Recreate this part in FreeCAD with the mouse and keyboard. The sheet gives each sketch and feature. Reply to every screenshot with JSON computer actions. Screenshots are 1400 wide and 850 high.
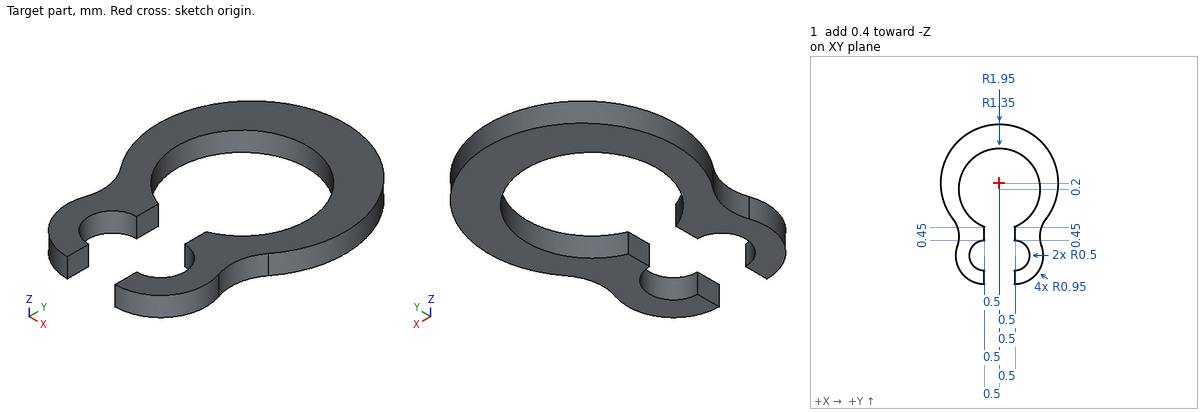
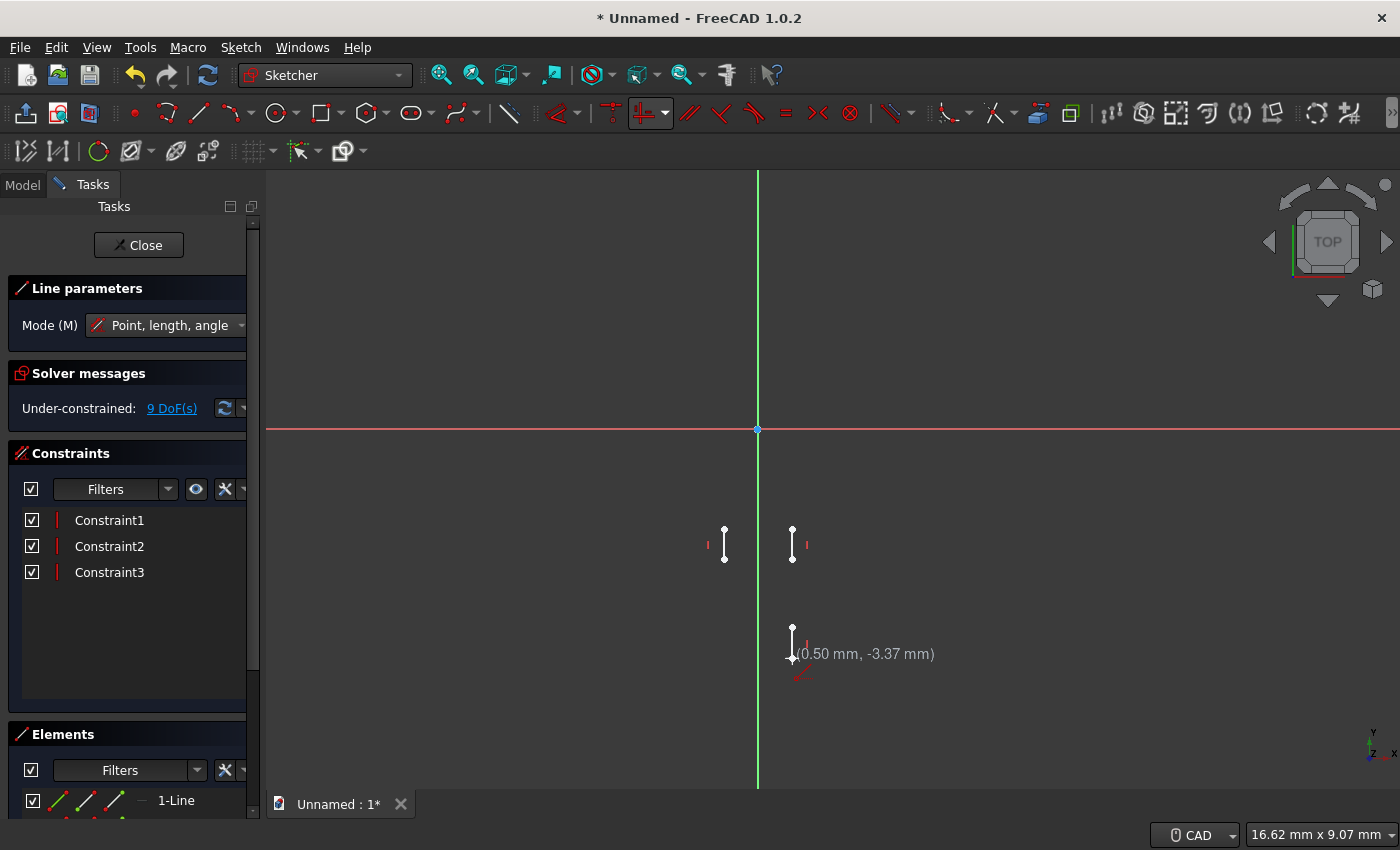
{"action": "left_click", "coordinate": [724, 658]}
{"action": "left_click", "coordinate": [724, 627]}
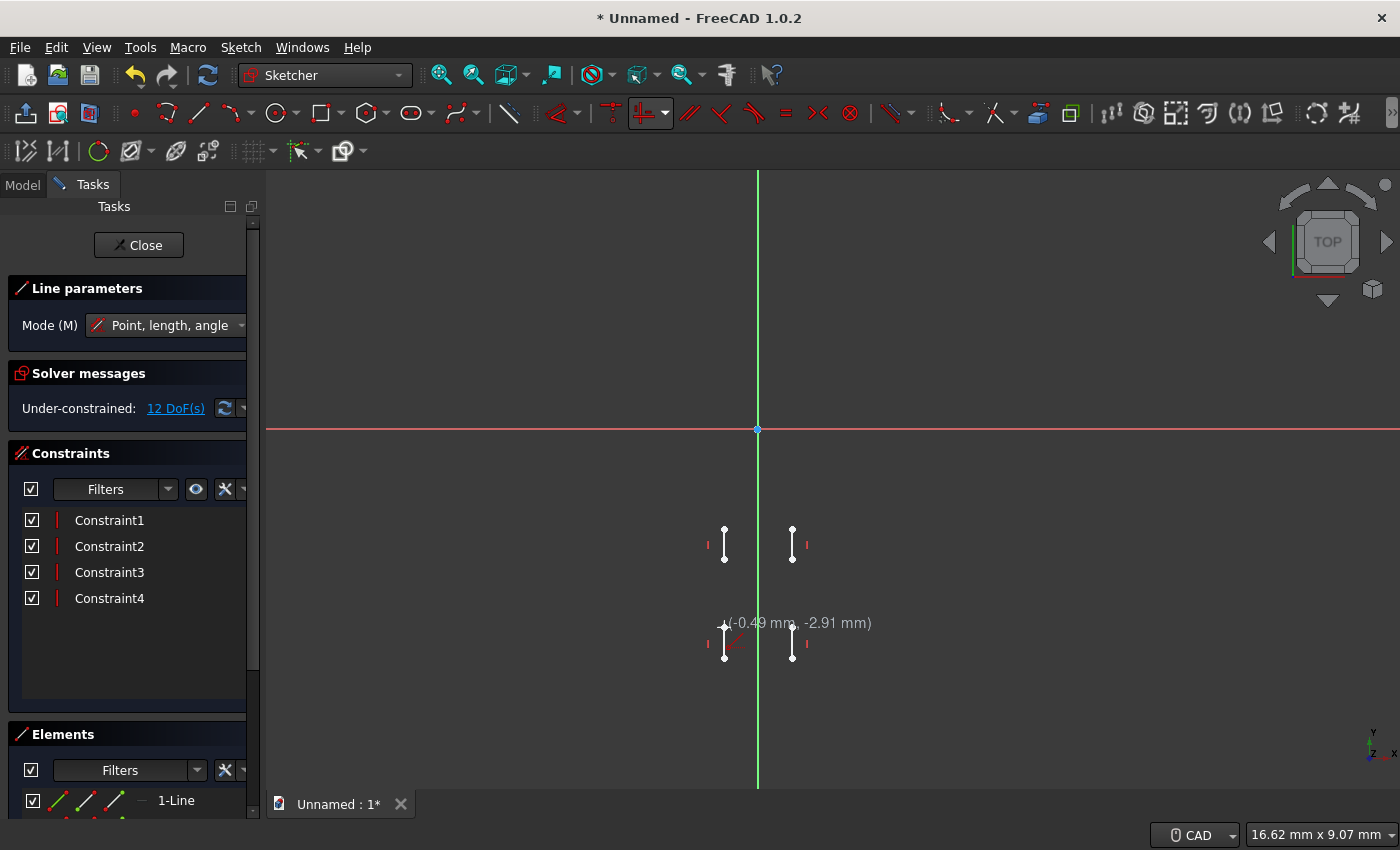
{"action": "left_click", "coordinate": [232, 114]}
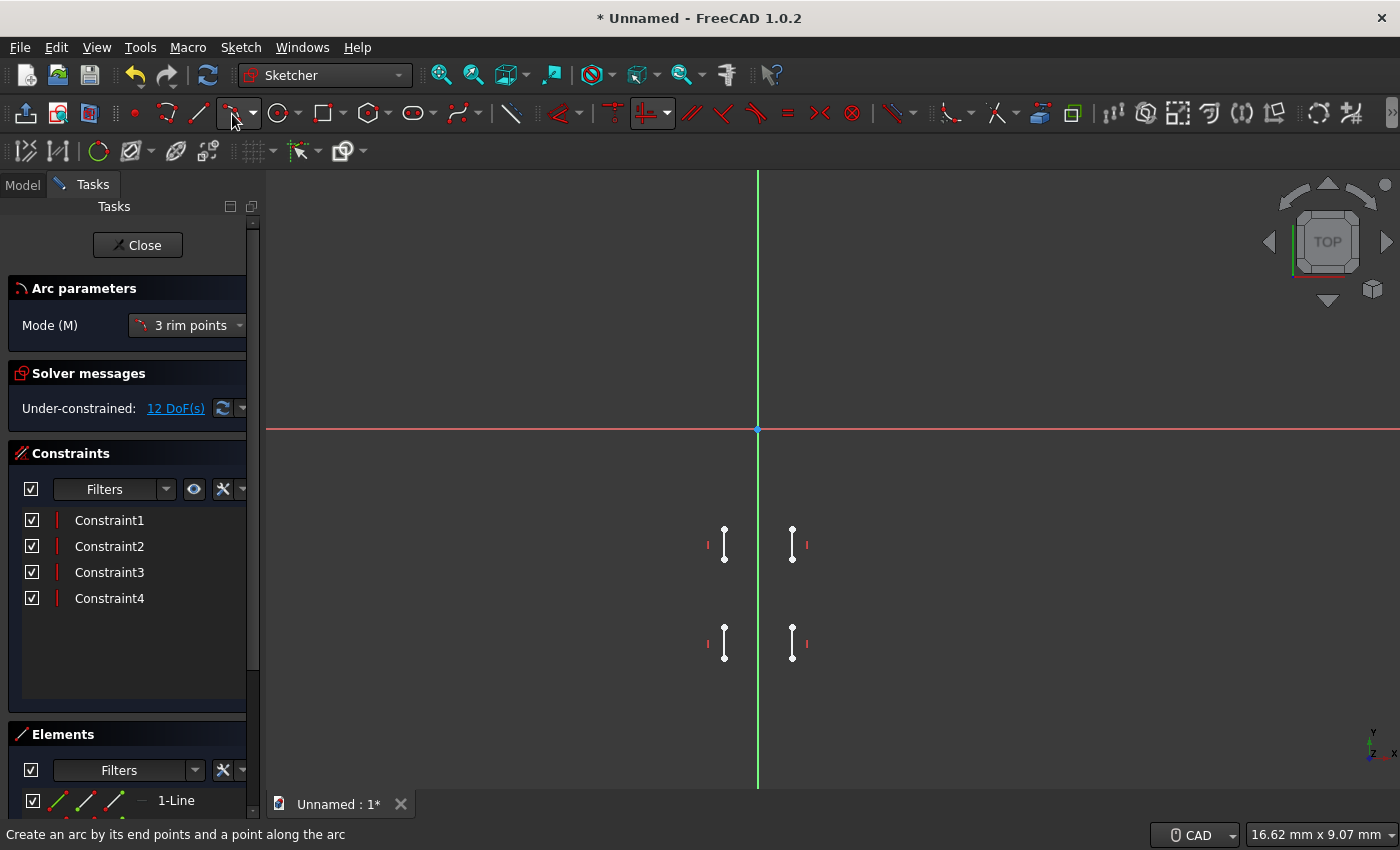
{"action": "left_click", "coordinate": [724, 530]}
{"action": "left_click", "coordinate": [792, 530]}
{"action": "left_click", "coordinate": [806, 365]}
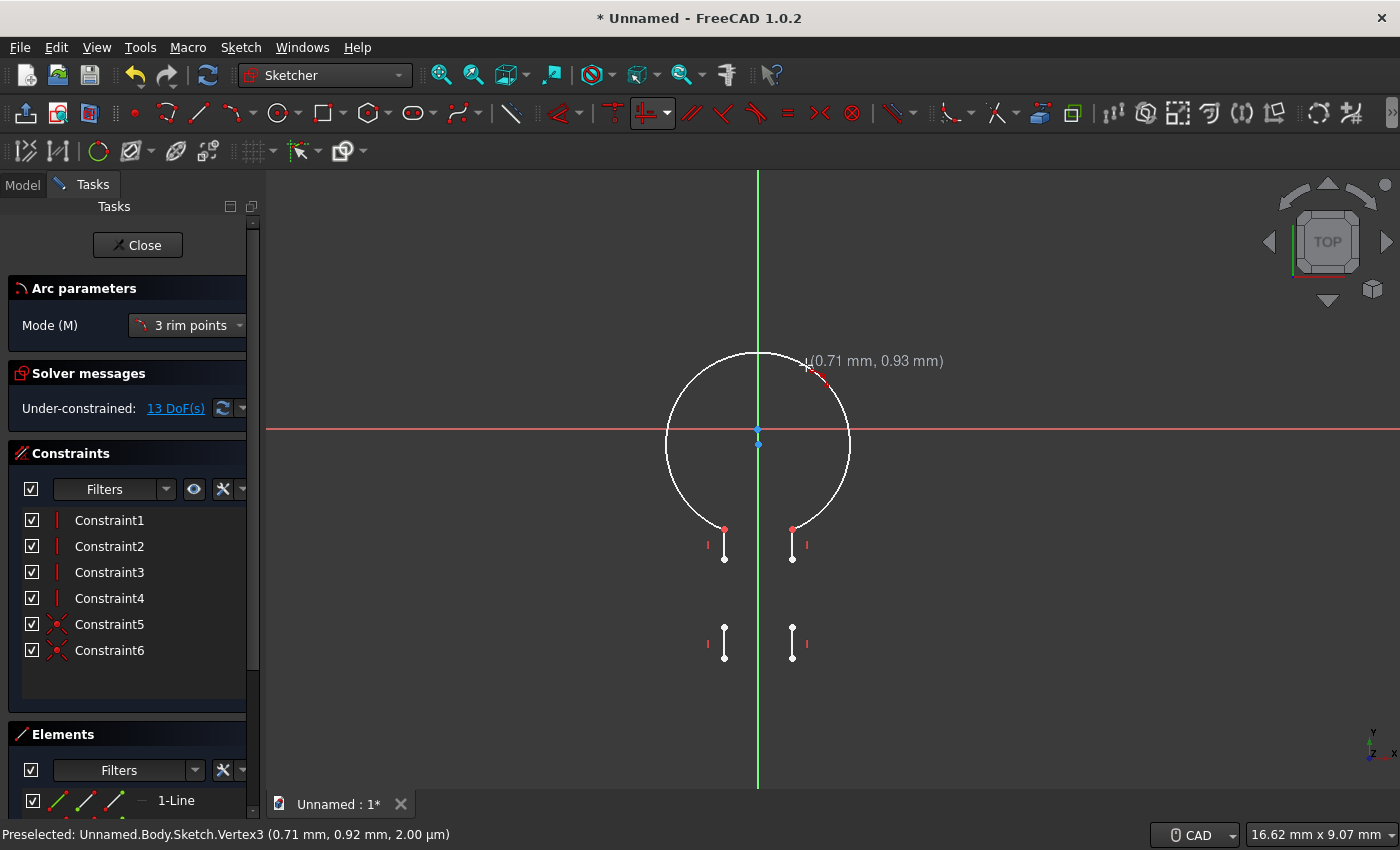
{"action": "left_click", "coordinate": [792, 560]}
{"action": "left_click", "coordinate": [792, 628]}
{"action": "left_click", "coordinate": [826, 593]}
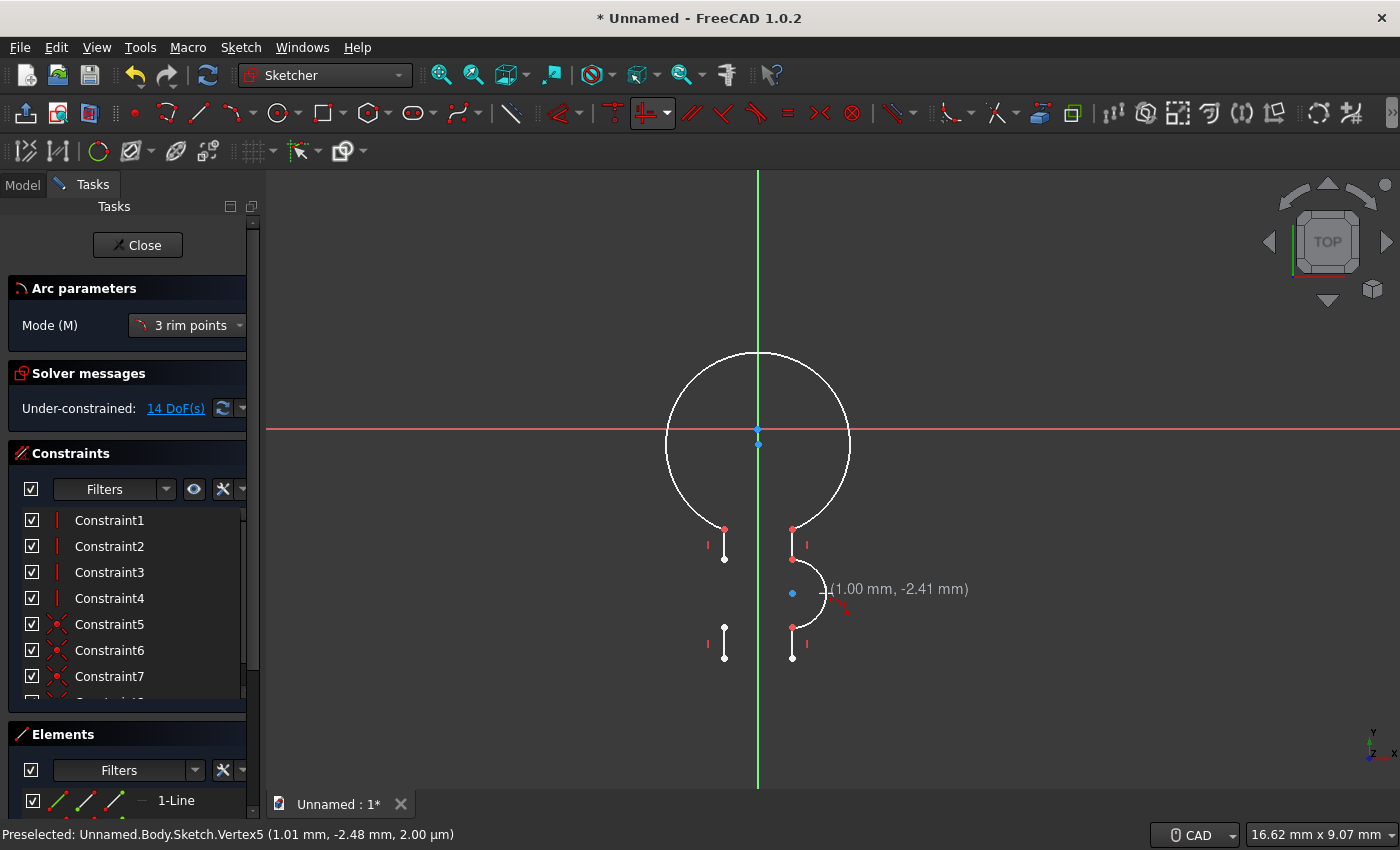
{"action": "left_click", "coordinate": [792, 659]}
{"action": "left_click", "coordinate": [853, 572]}
{"action": "left_click", "coordinate": [845, 631]}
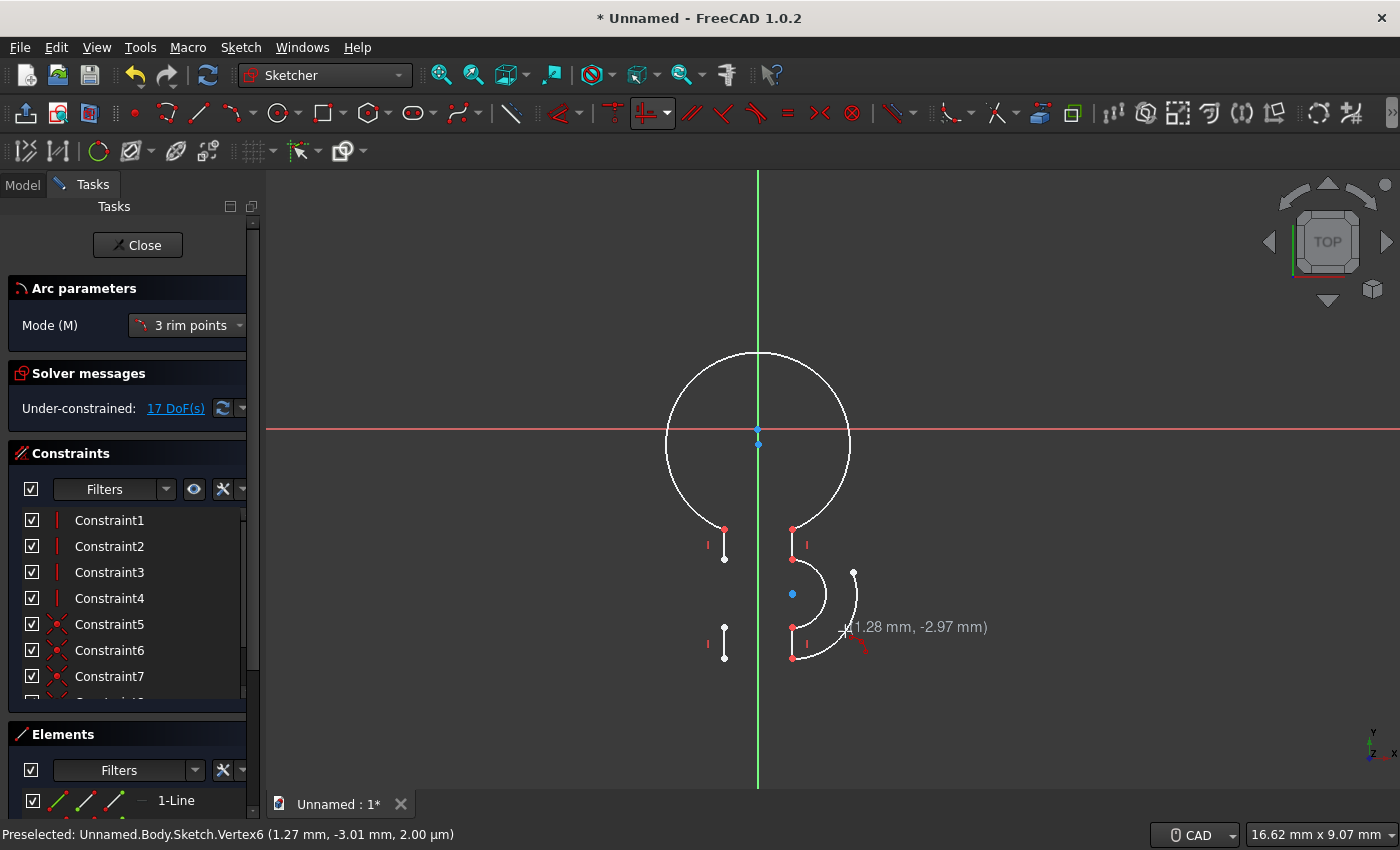
{"action": "left_click", "coordinate": [853, 573]}
{"action": "left_click", "coordinate": [863, 511]}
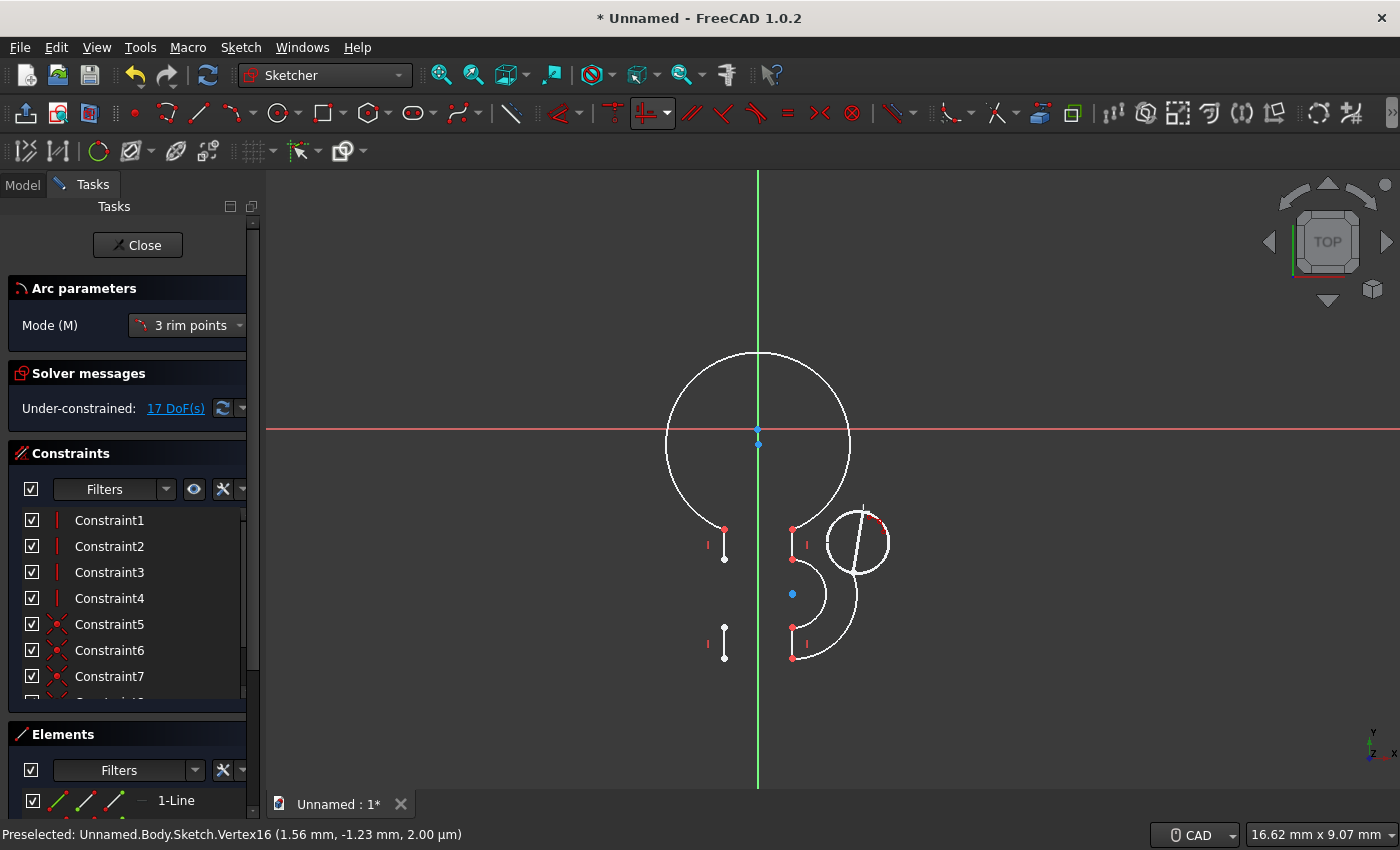
{"action": "scroll", "coordinate": [850, 540], "scroll_direction": "up", "scroll_amount": 4}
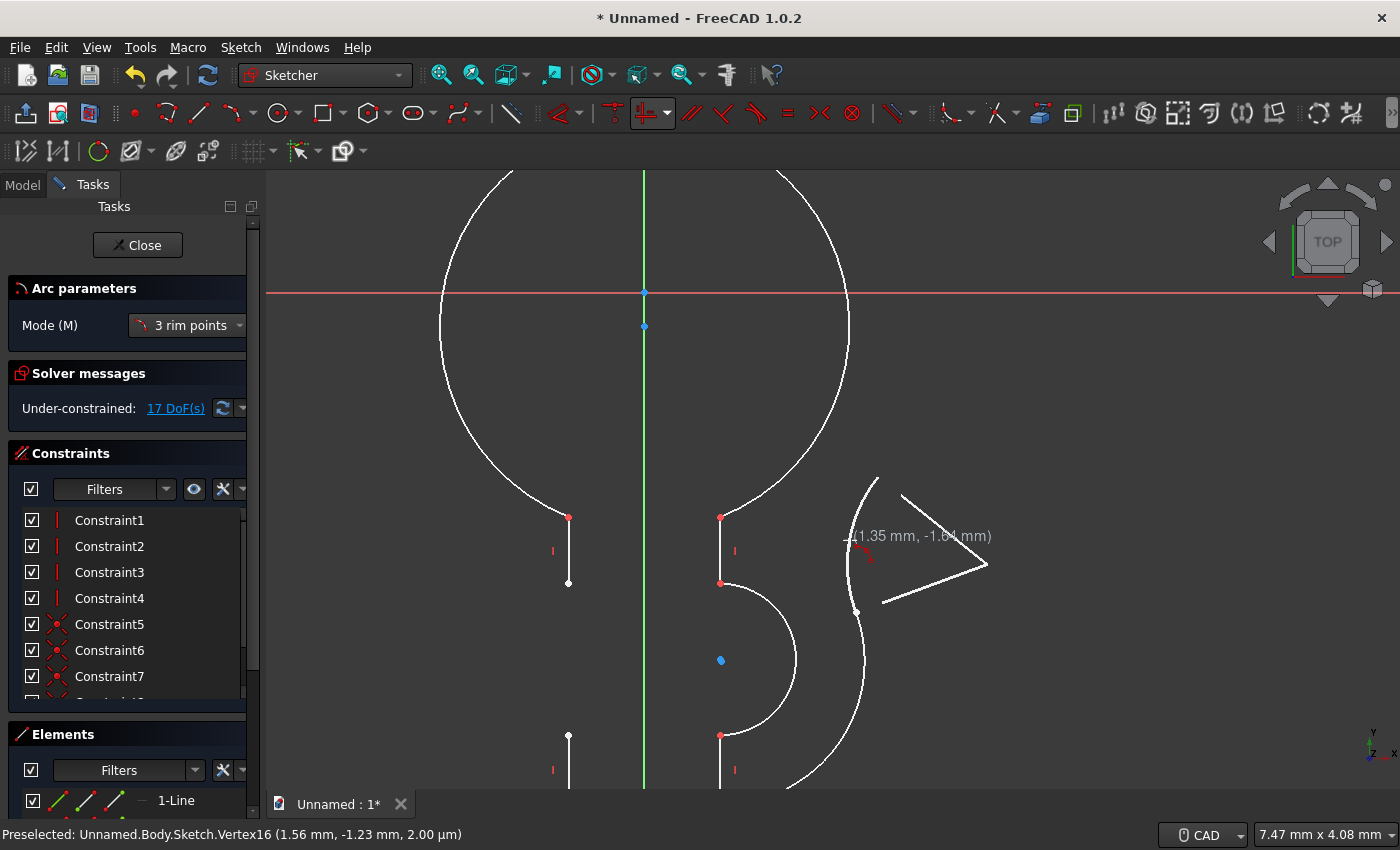
{"action": "left_click", "coordinate": [850, 539]}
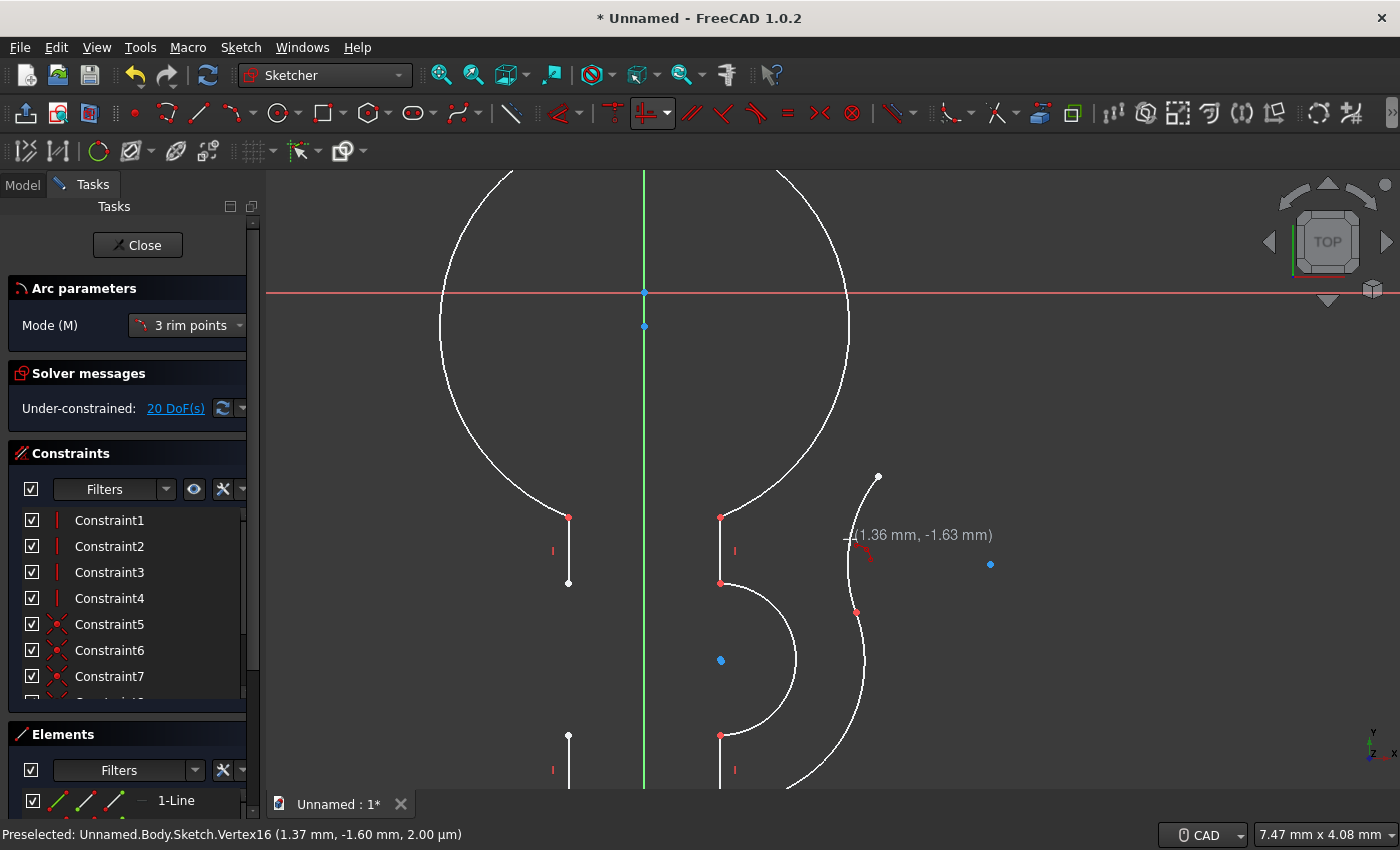
{"action": "left_click", "coordinate": [878, 477]}
{"action": "left_click", "coordinate": [410, 474]}